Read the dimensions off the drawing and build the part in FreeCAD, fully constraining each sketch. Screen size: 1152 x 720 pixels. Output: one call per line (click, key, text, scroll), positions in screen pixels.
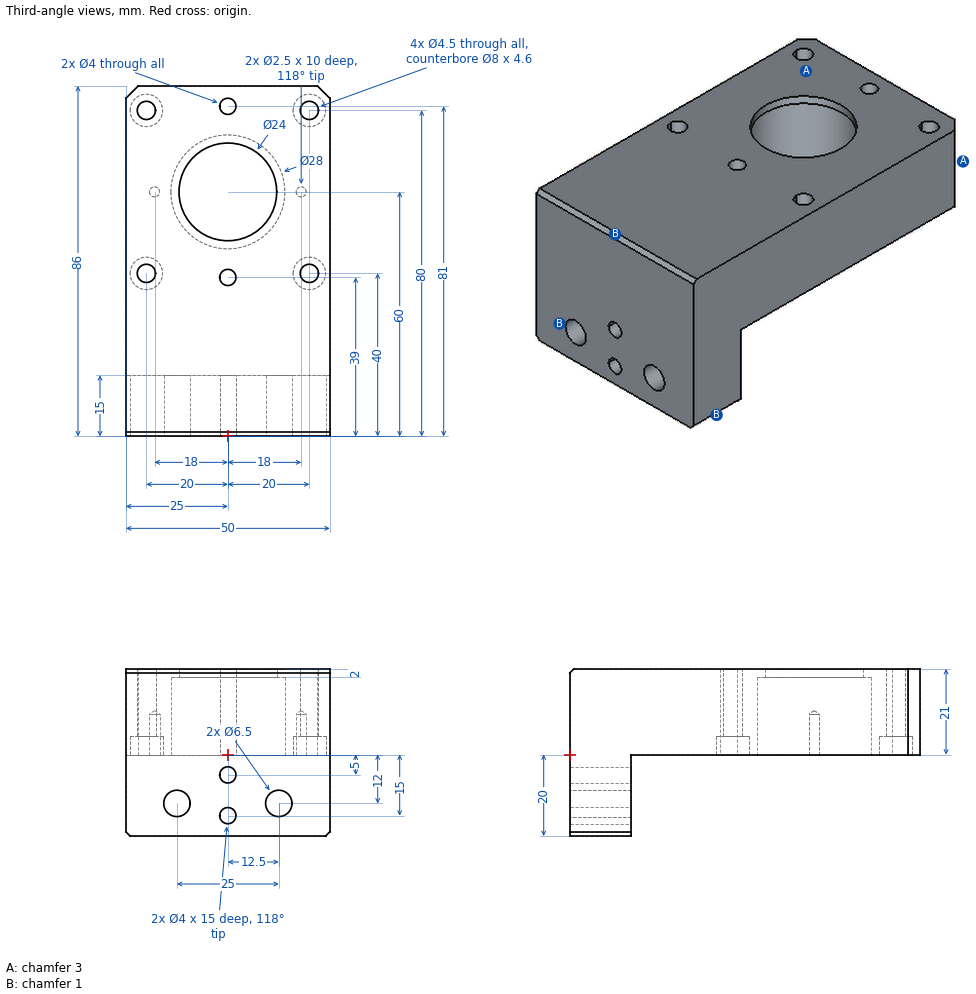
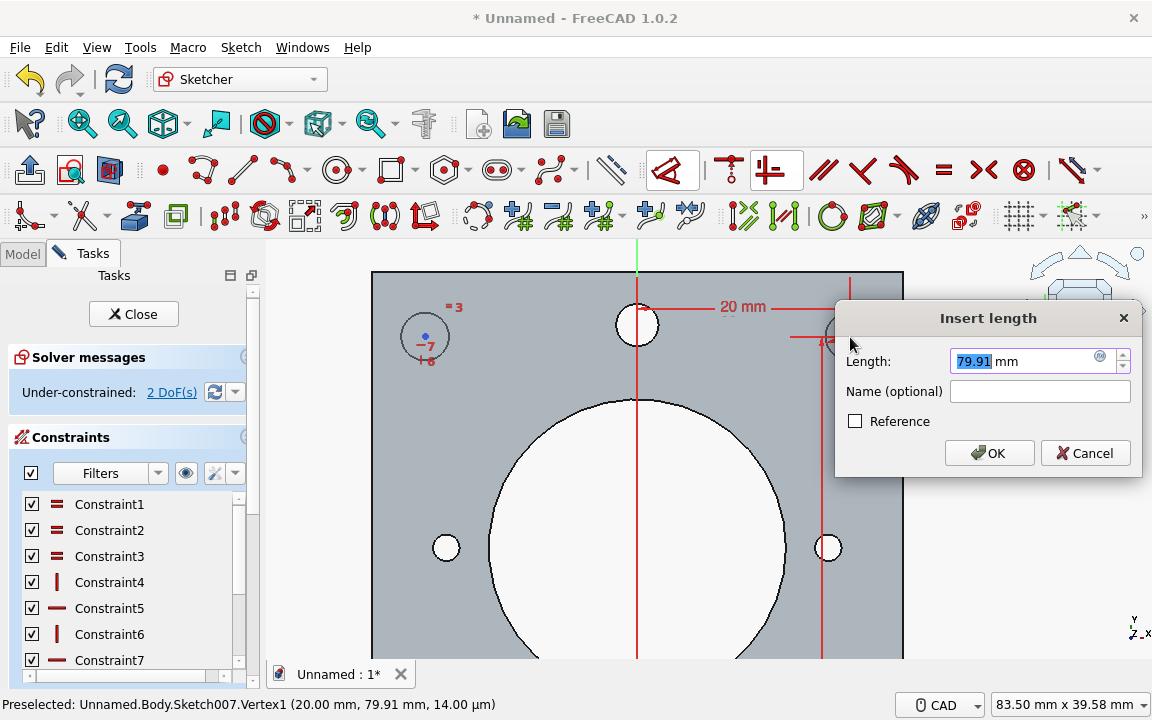
text(80)
key(Return)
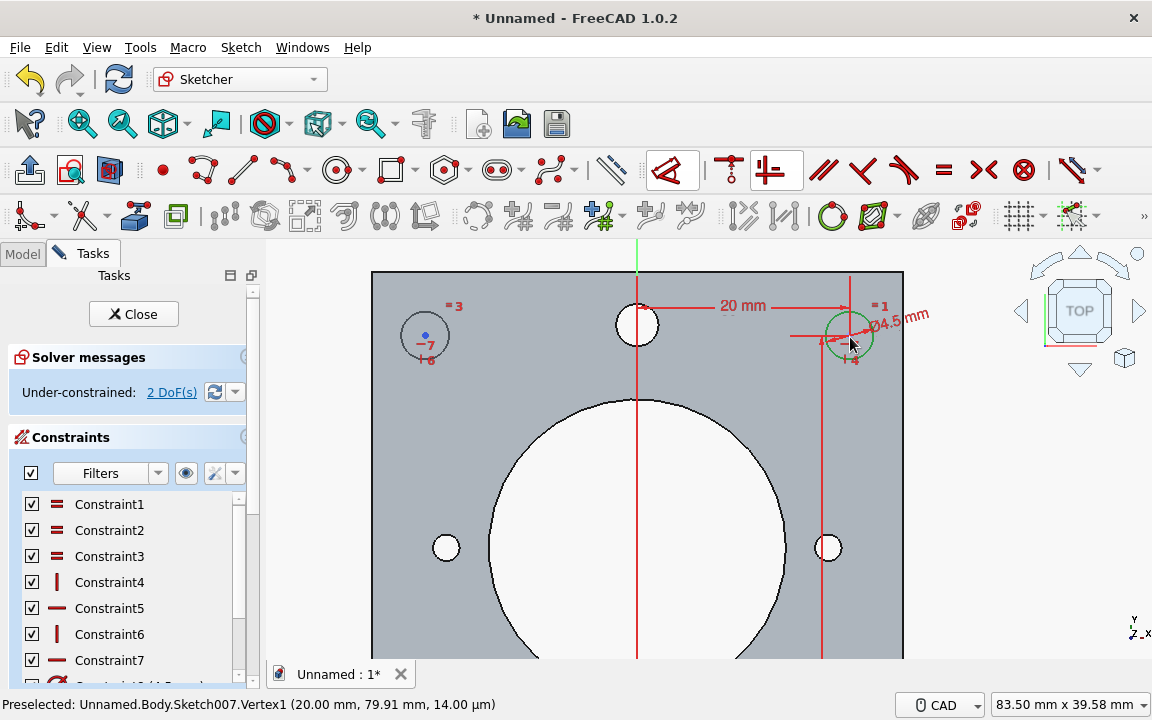
scroll(642, 320, down, 6)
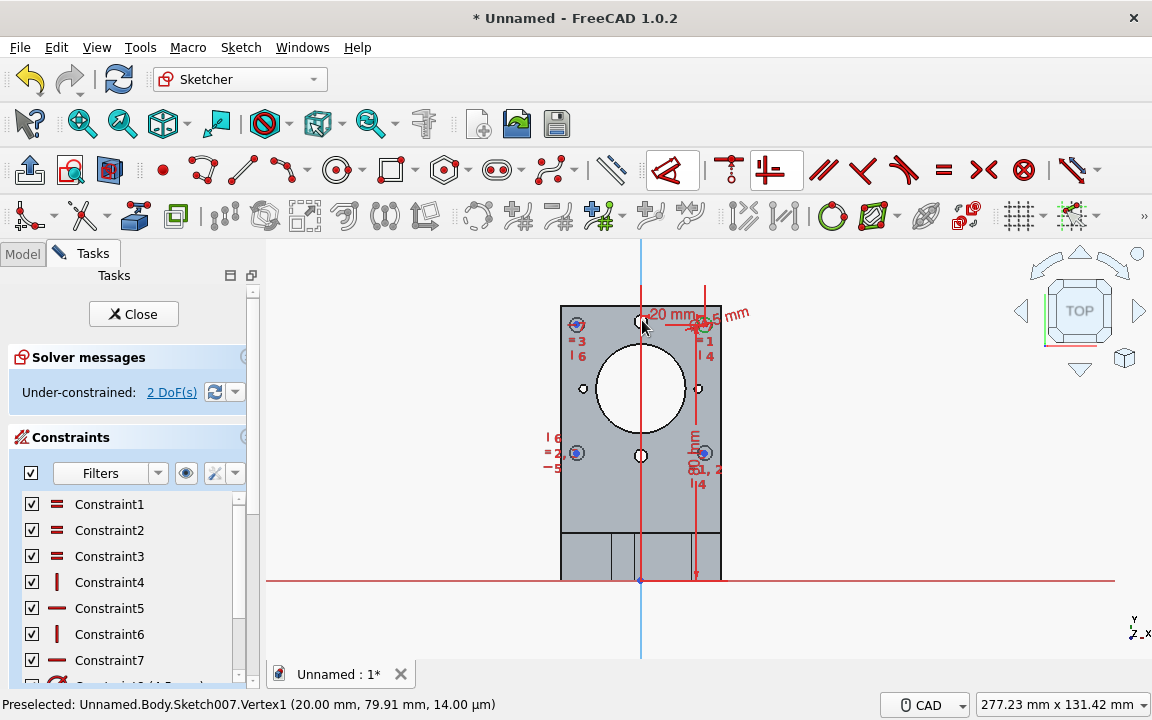
click(705, 453)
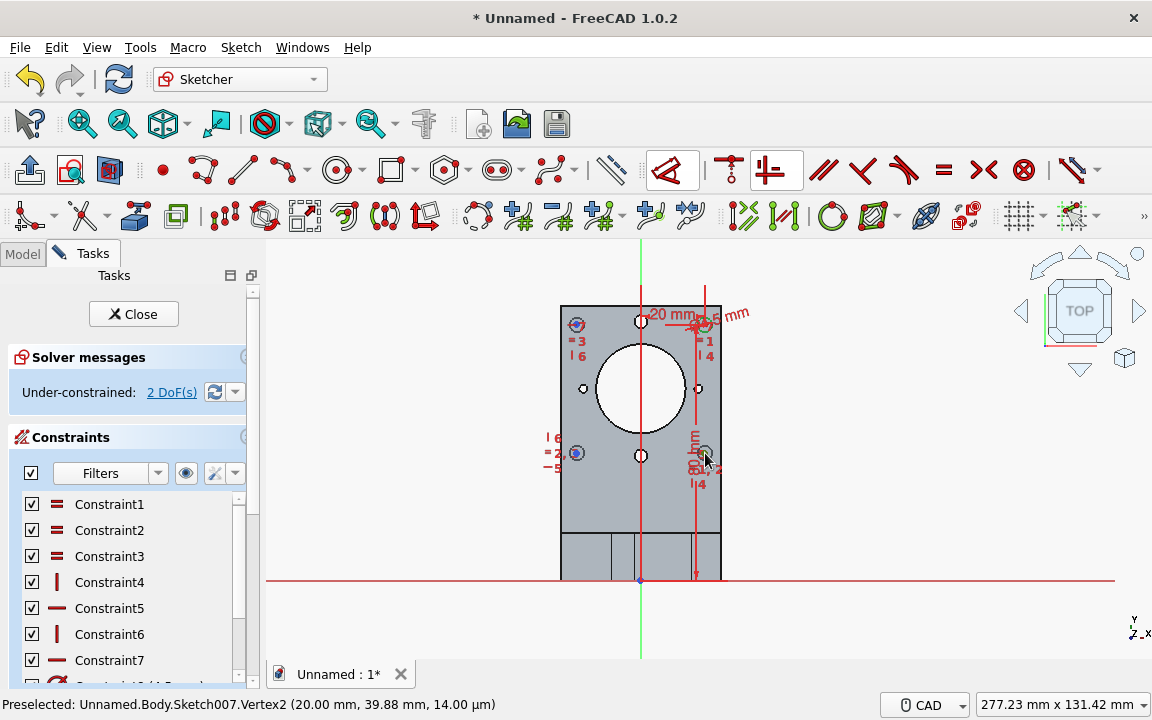
key(i)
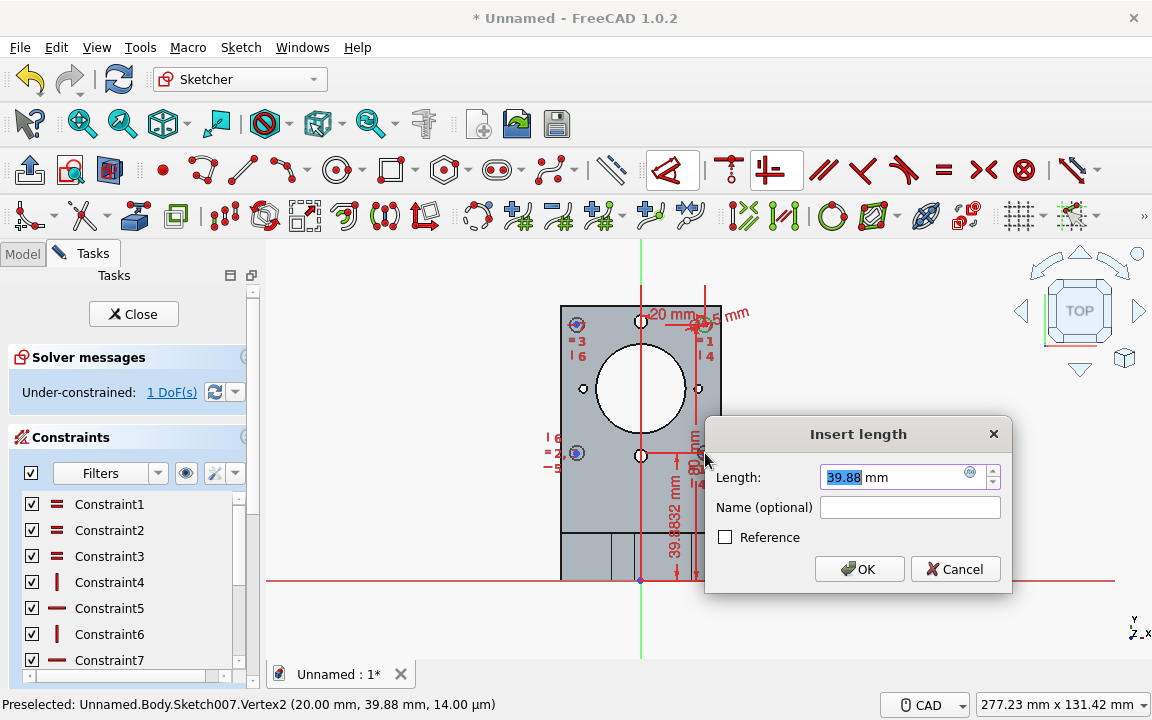
text(40)
key(Return)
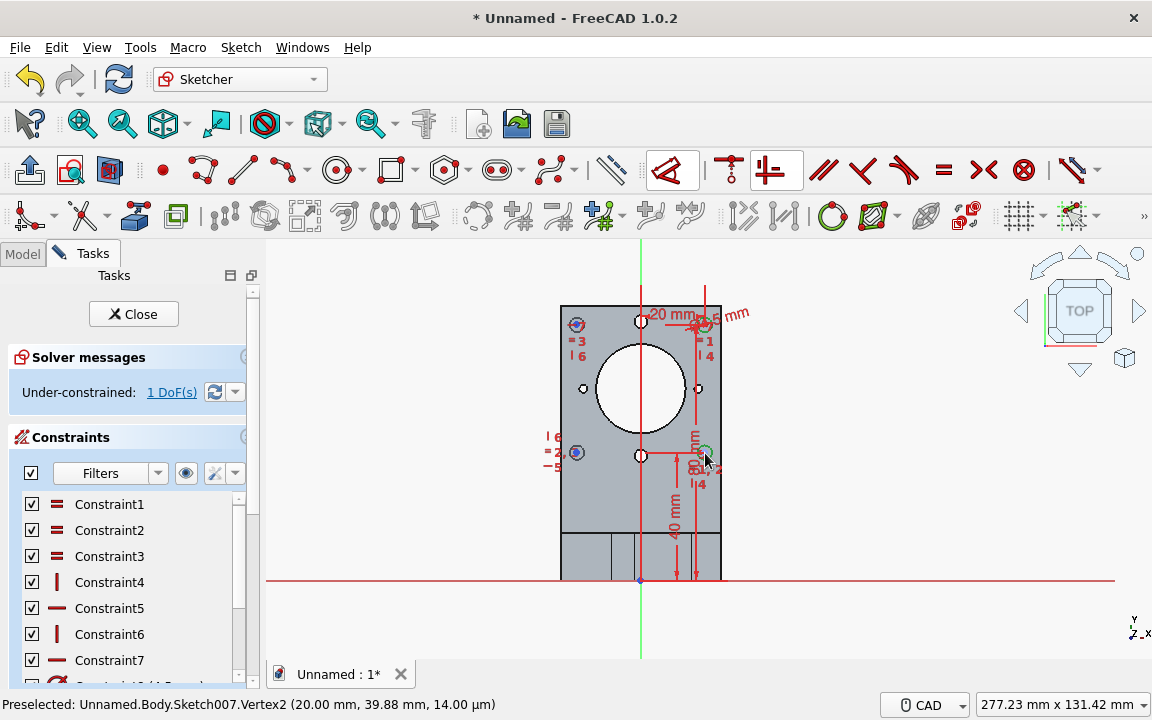
click(577, 453)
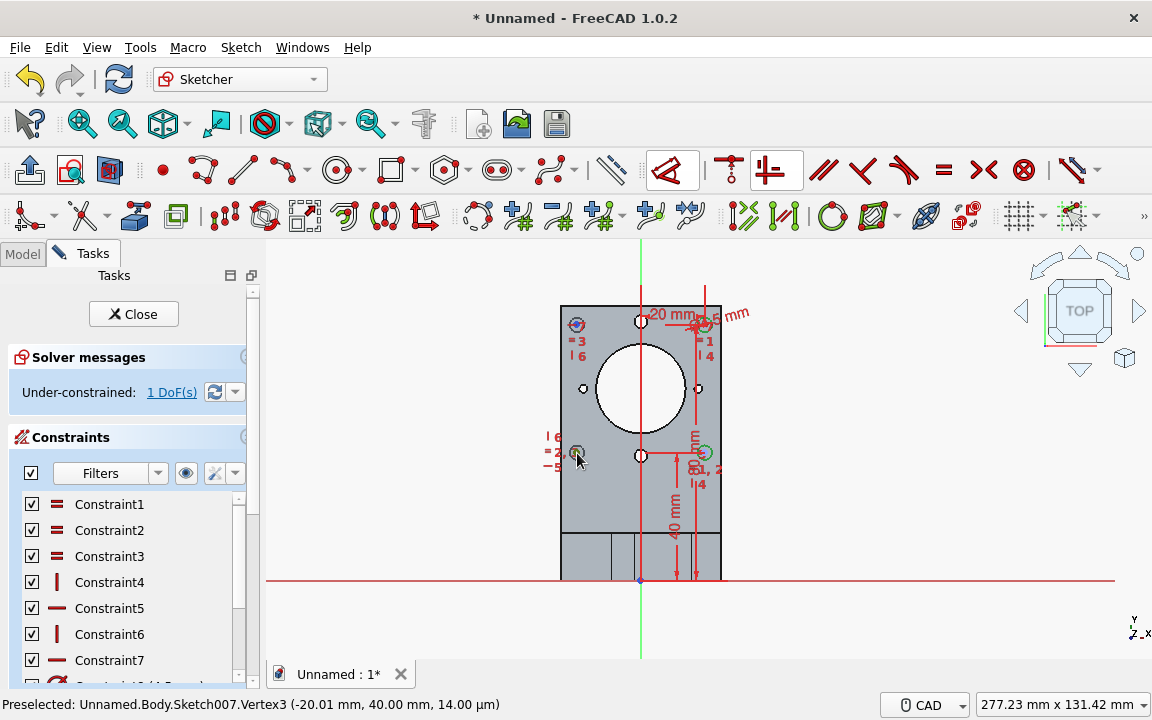
key(l)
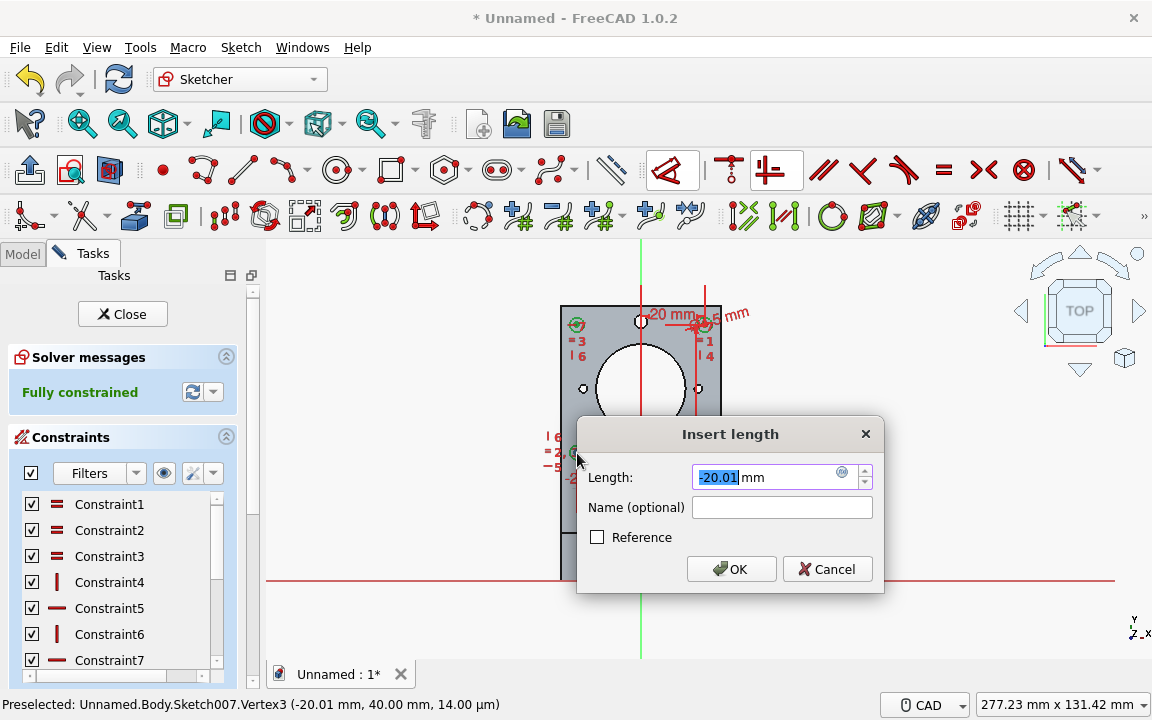
text(-20)
key(Return)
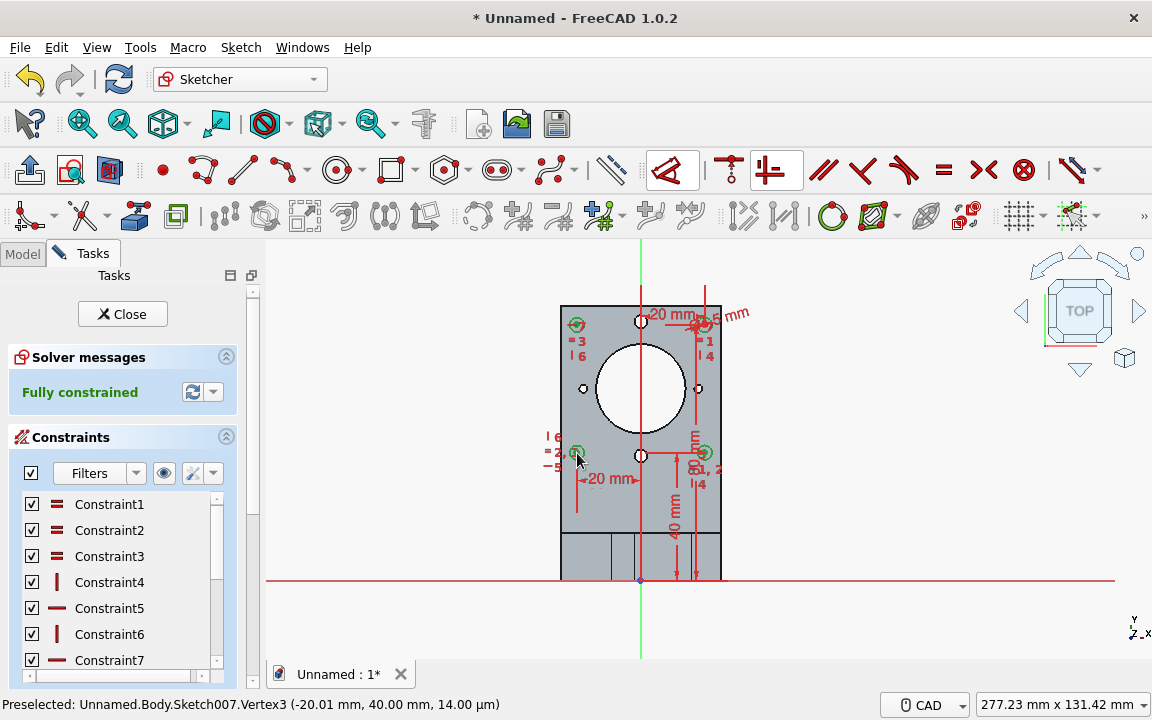
click(123, 314)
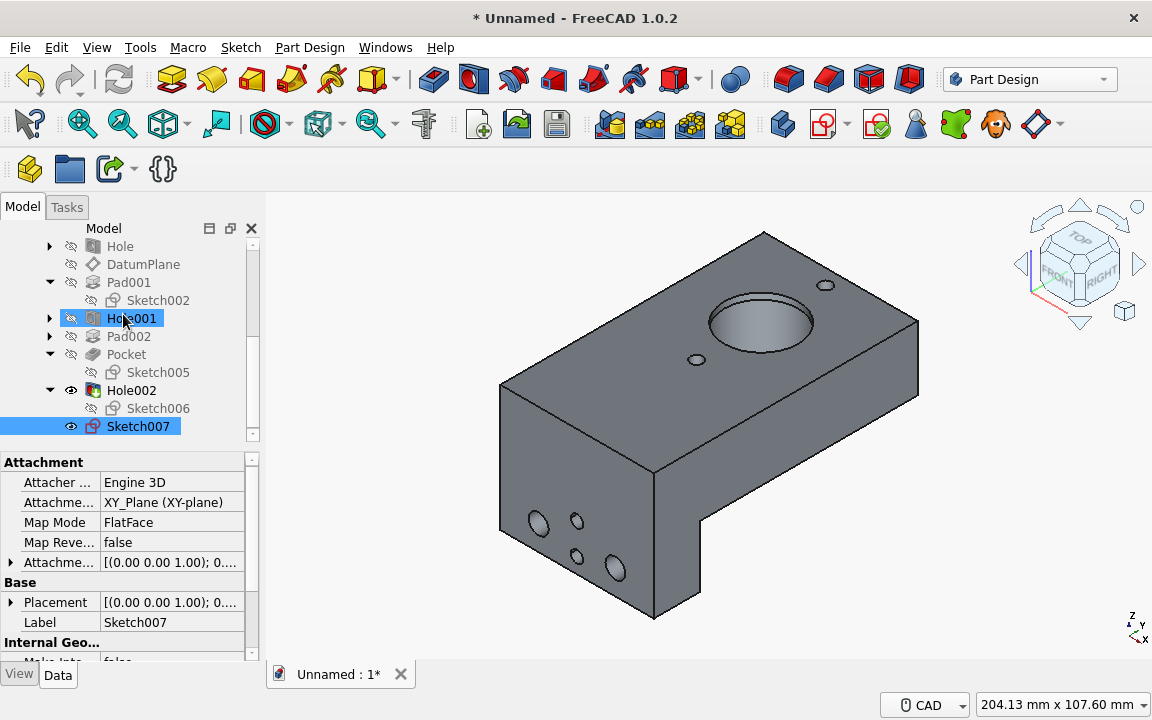
click(474, 80)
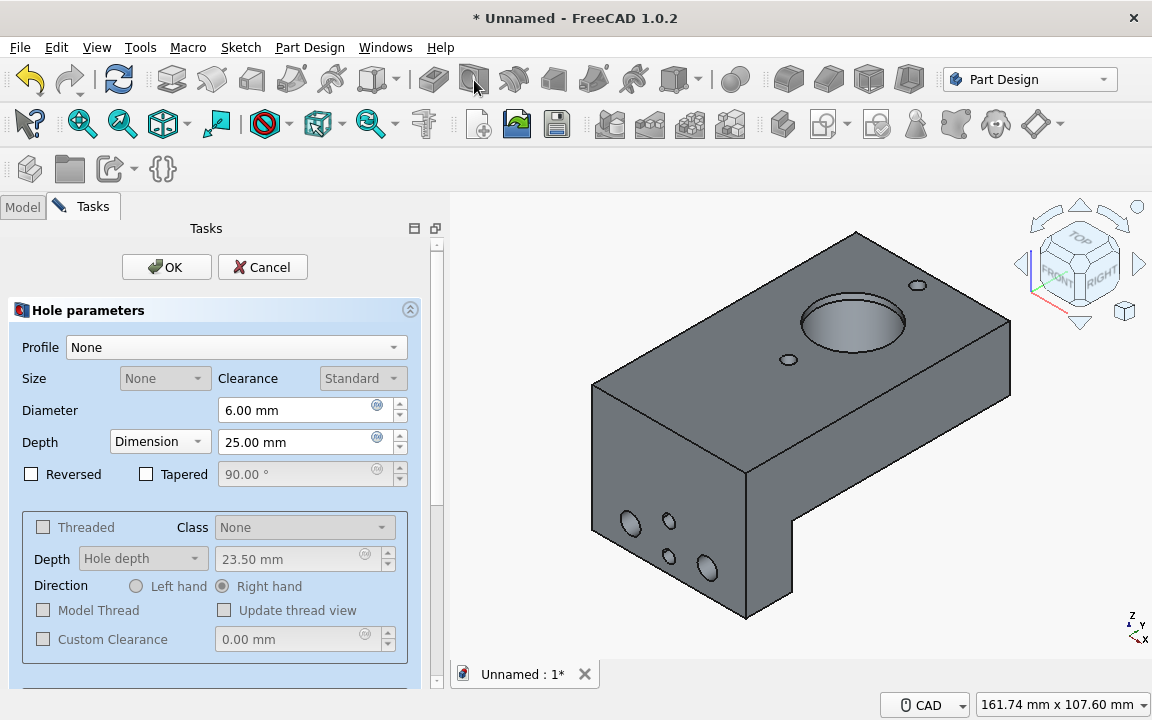
triple_click(305, 410)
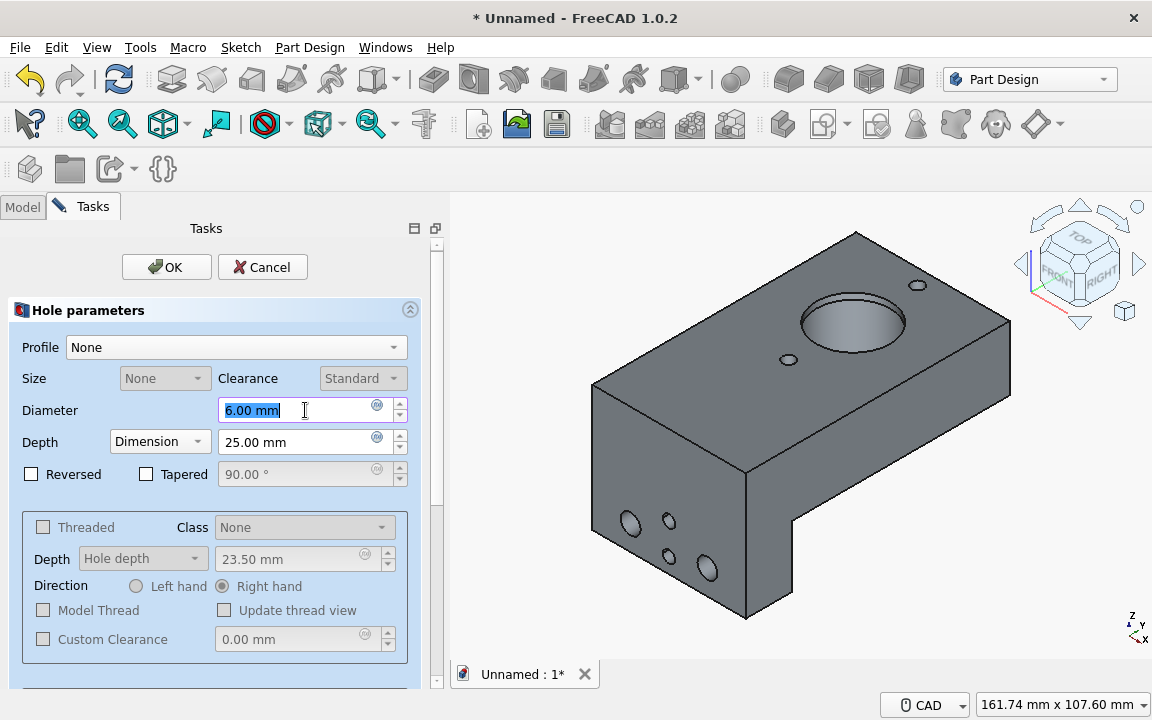
text(4.5)
key(Tab)